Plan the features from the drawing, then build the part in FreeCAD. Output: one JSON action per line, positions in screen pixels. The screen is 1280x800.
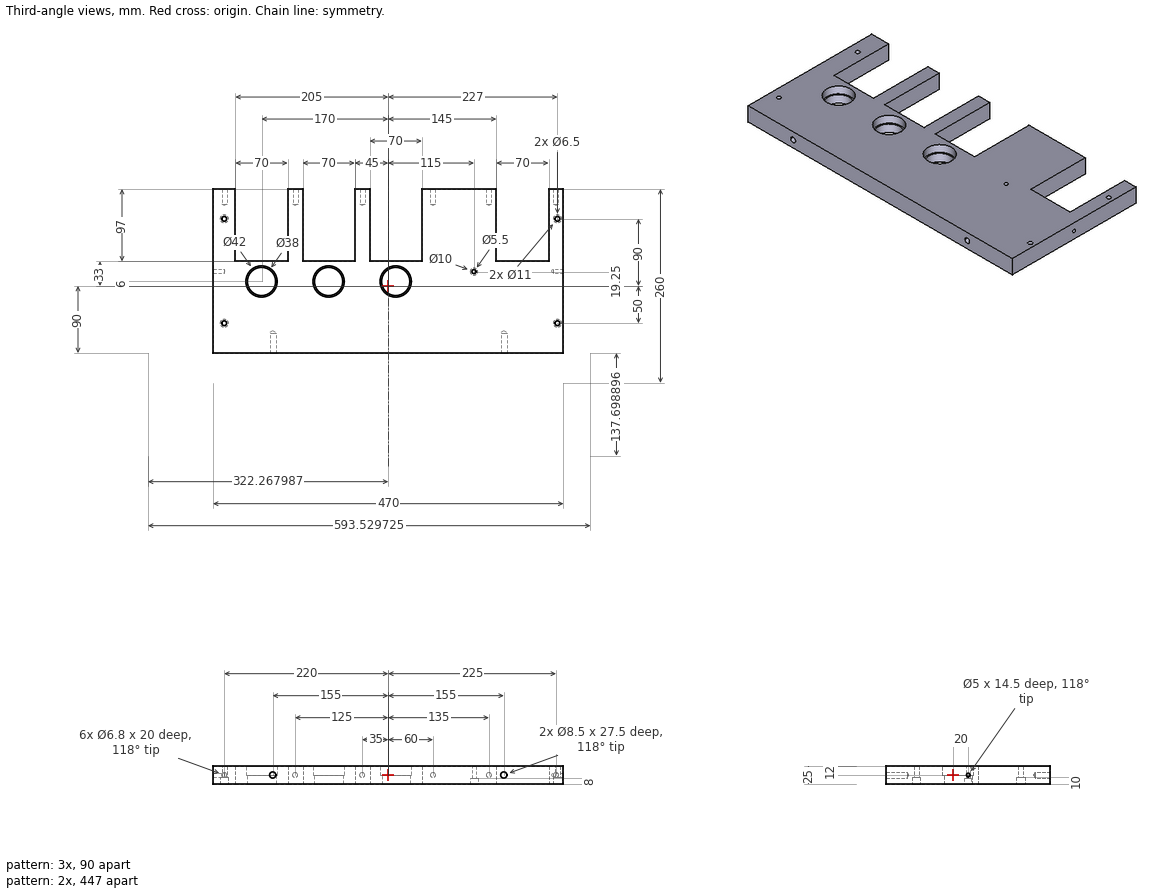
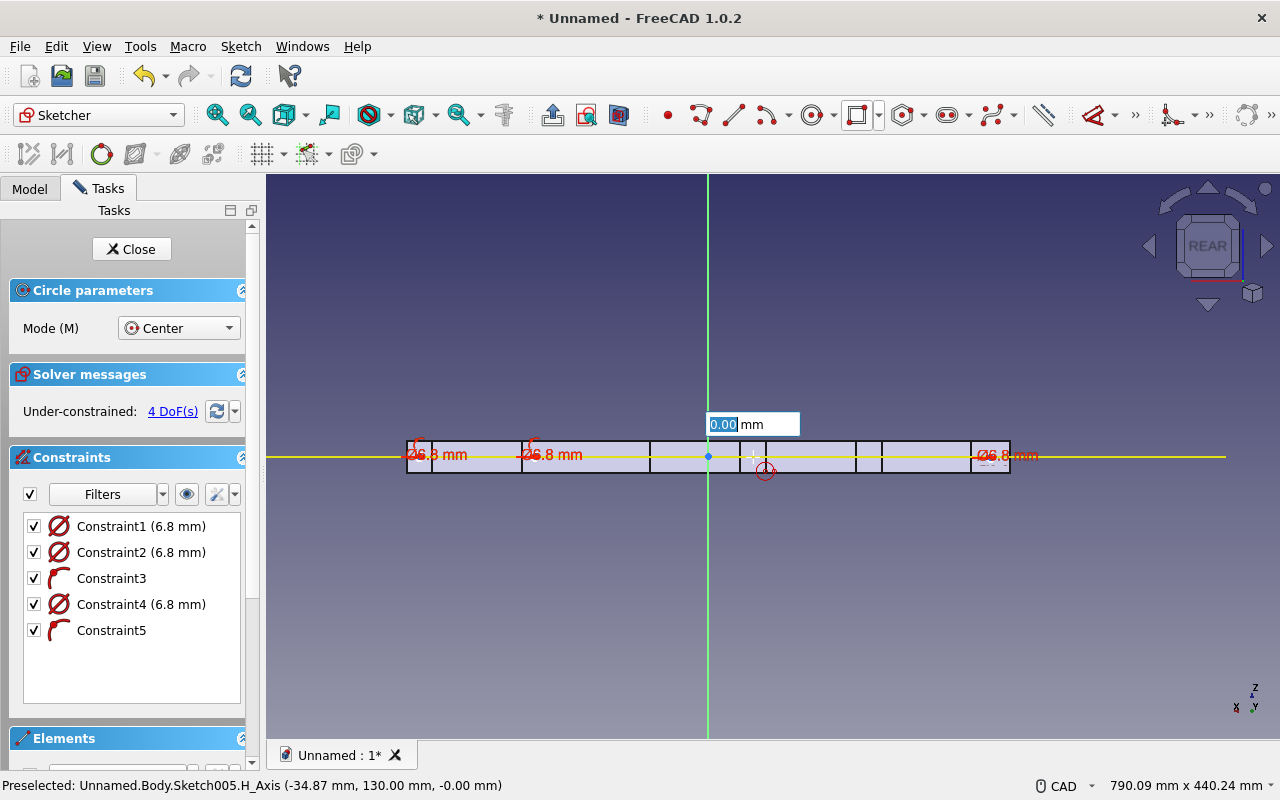
{"action": "scroll", "coordinate": [752, 461], "scroll_direction": "up", "scroll_amount": 7}
{"action": "mouse_move", "coordinate": [749, 459]}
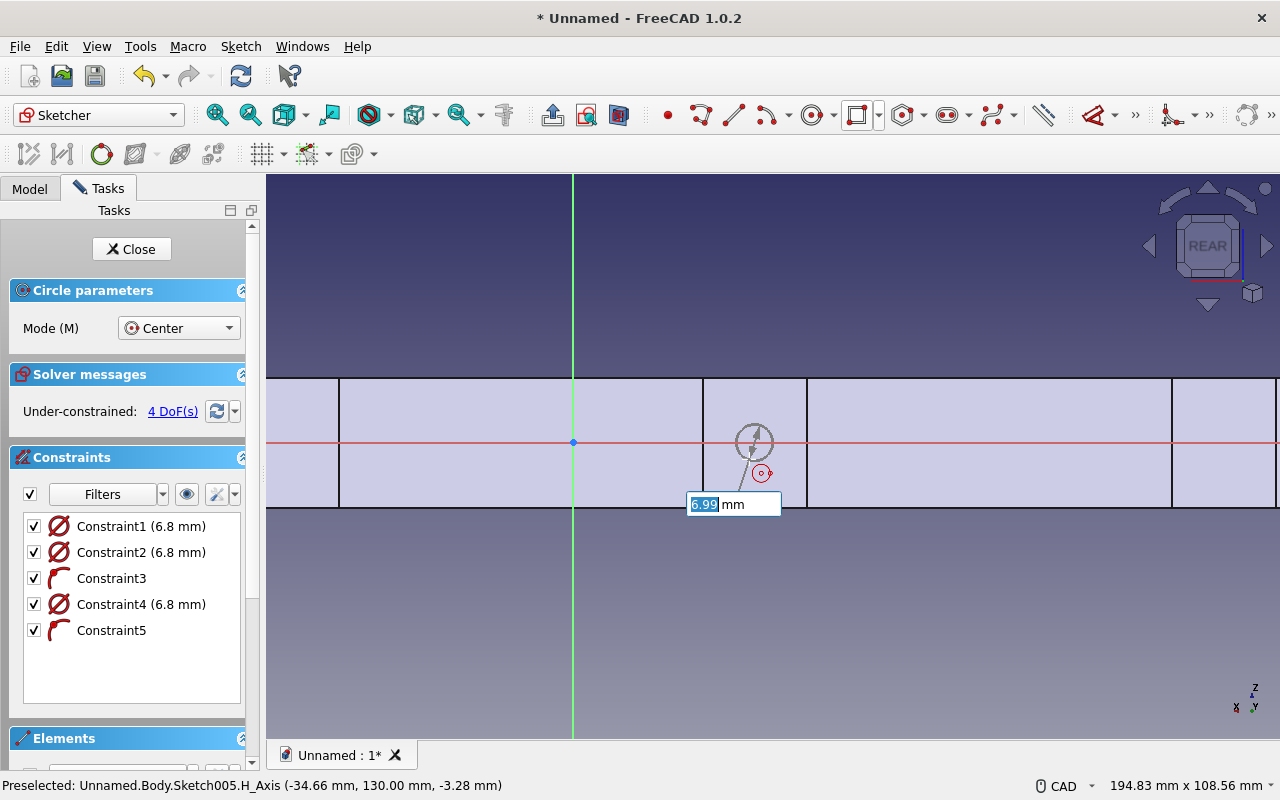
{"action": "type", "text": "6.8"}
{"action": "key", "text": "Return"}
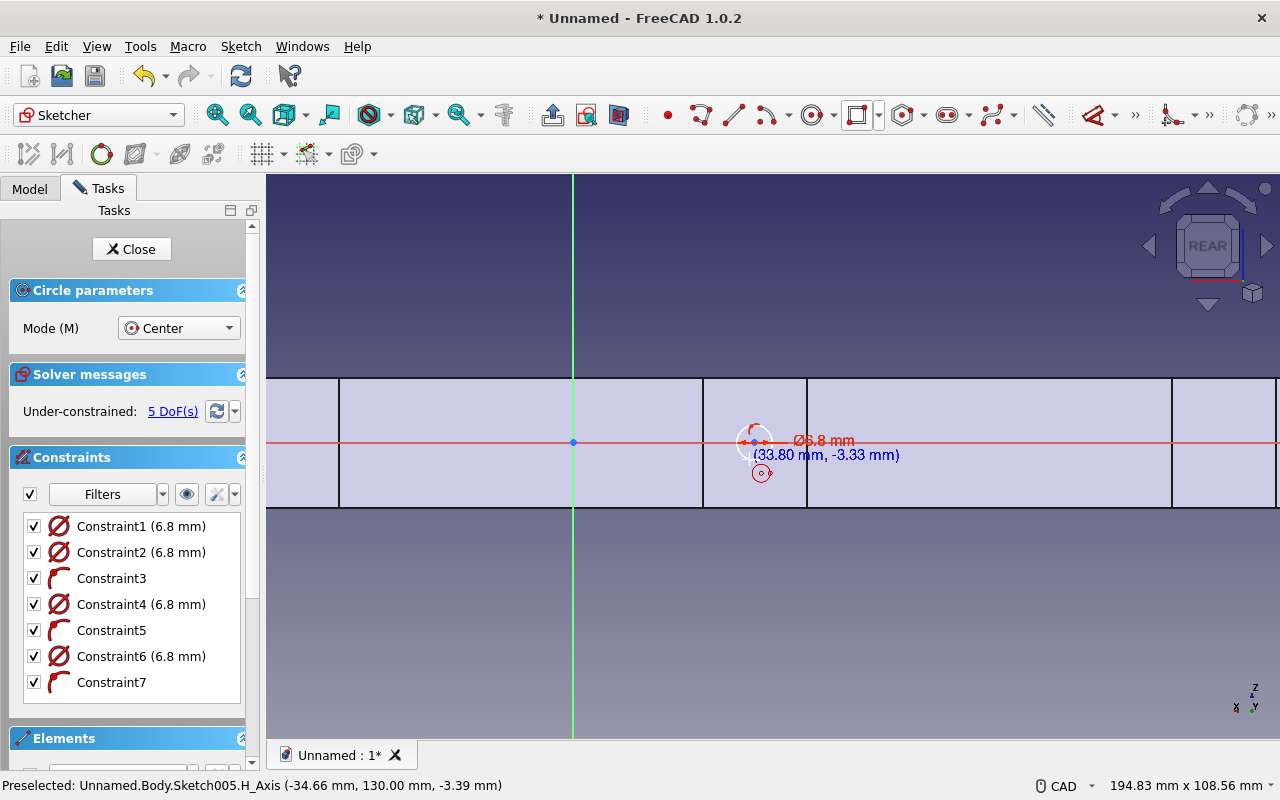
{"action": "scroll", "coordinate": [752, 461], "scroll_direction": "down", "scroll_amount": 7}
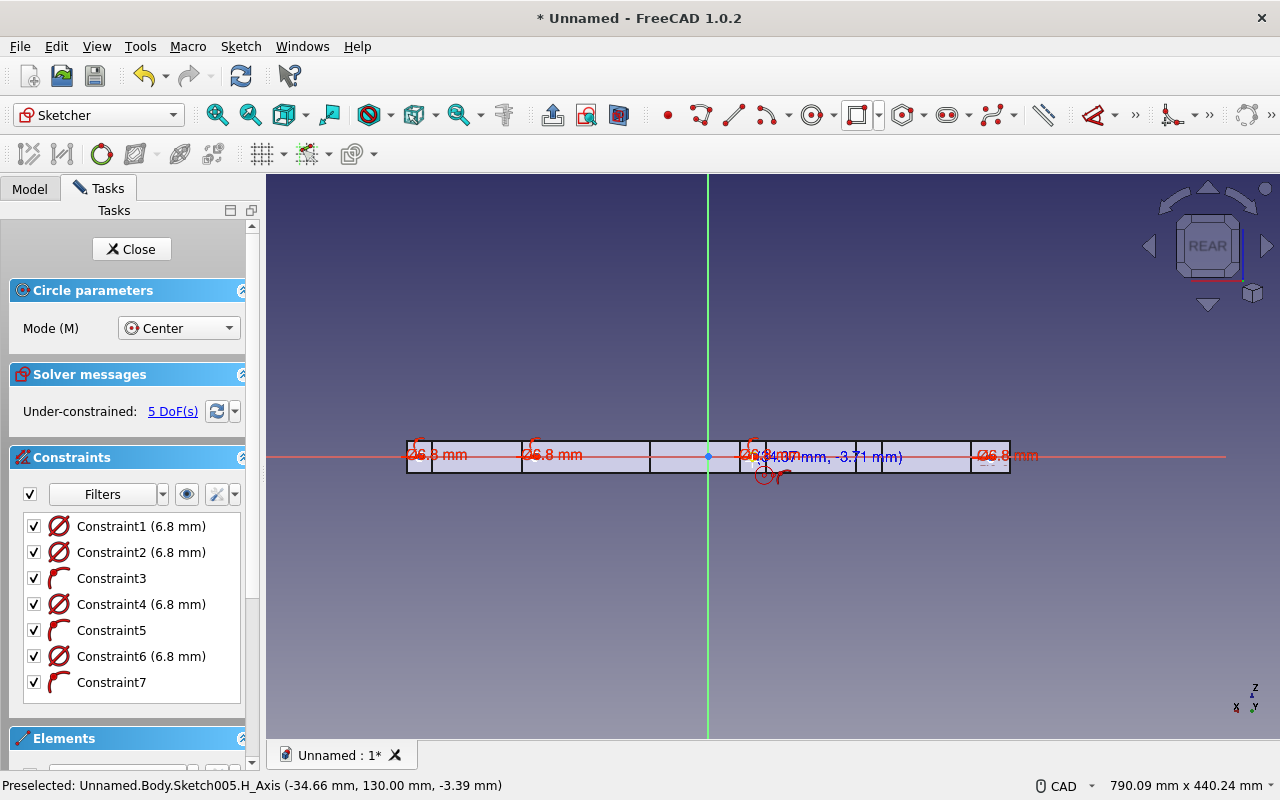
{"action": "scroll", "coordinate": [869, 457], "scroll_direction": "up", "scroll_amount": 9}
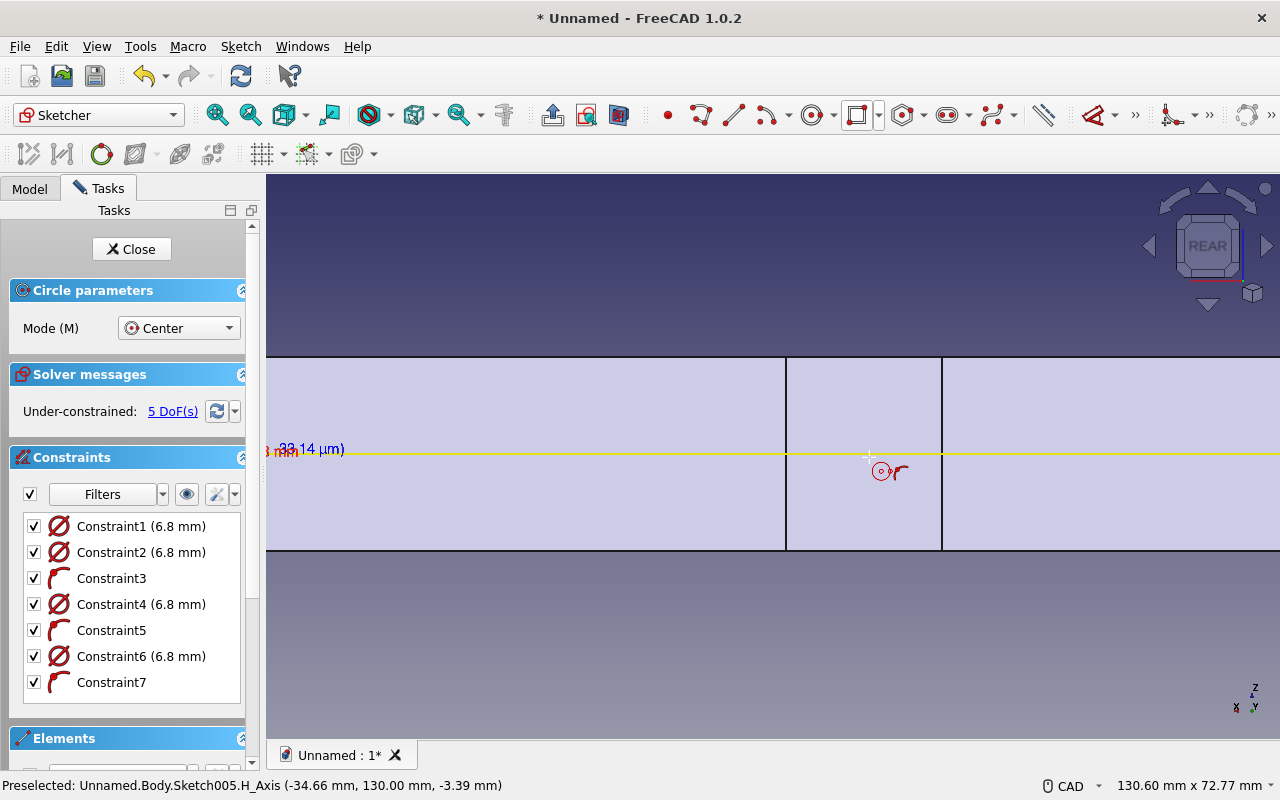
{"action": "scroll", "coordinate": [869, 457], "scroll_direction": "down", "scroll_amount": 9}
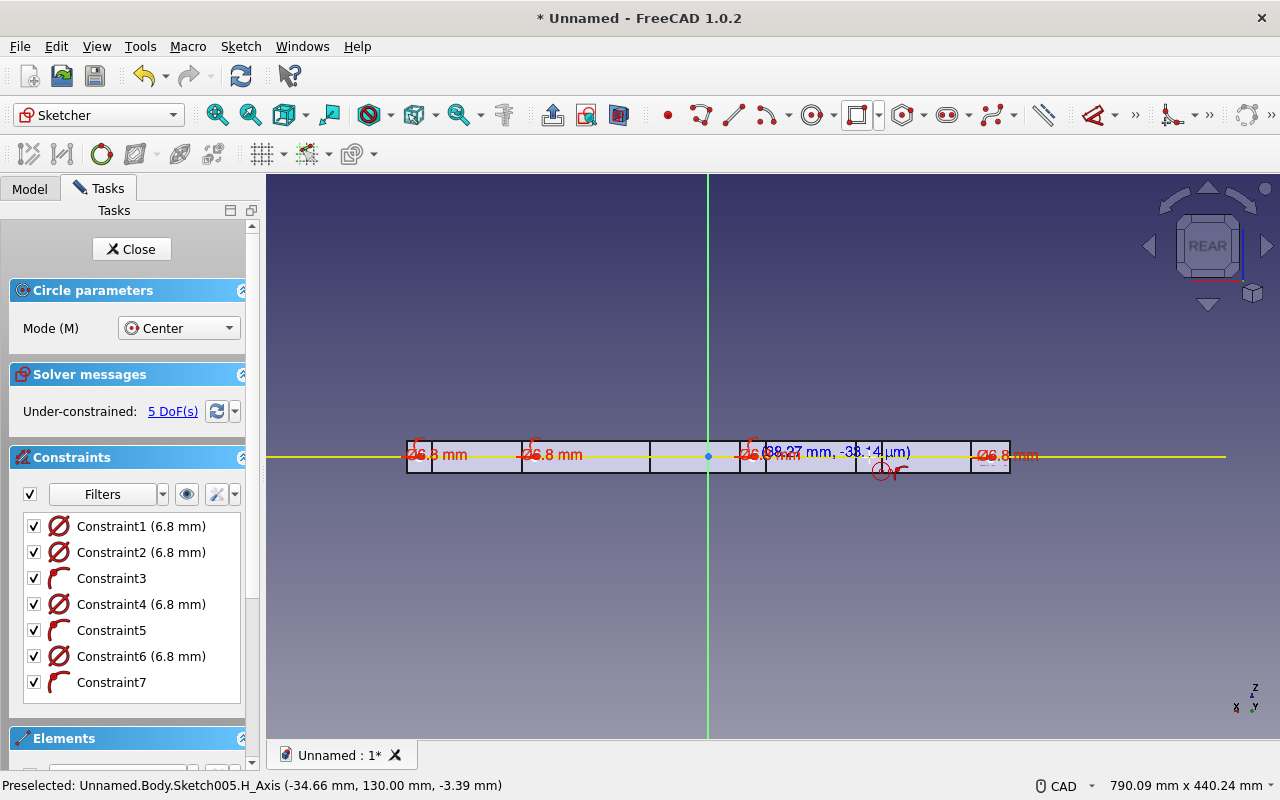
{"action": "left_click", "coordinate": [869, 457]}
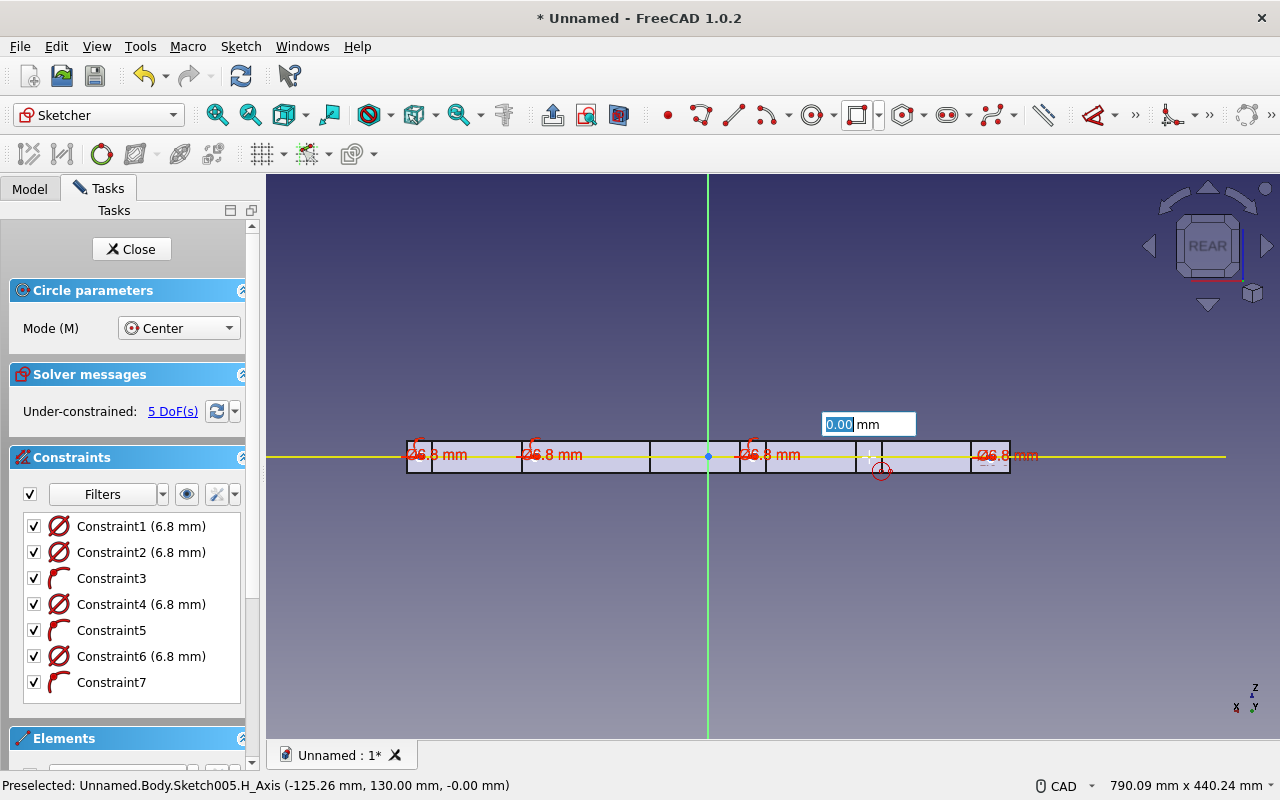
{"action": "scroll", "coordinate": [867, 461], "scroll_direction": "up", "scroll_amount": 7}
{"action": "mouse_move", "coordinate": [866, 459]}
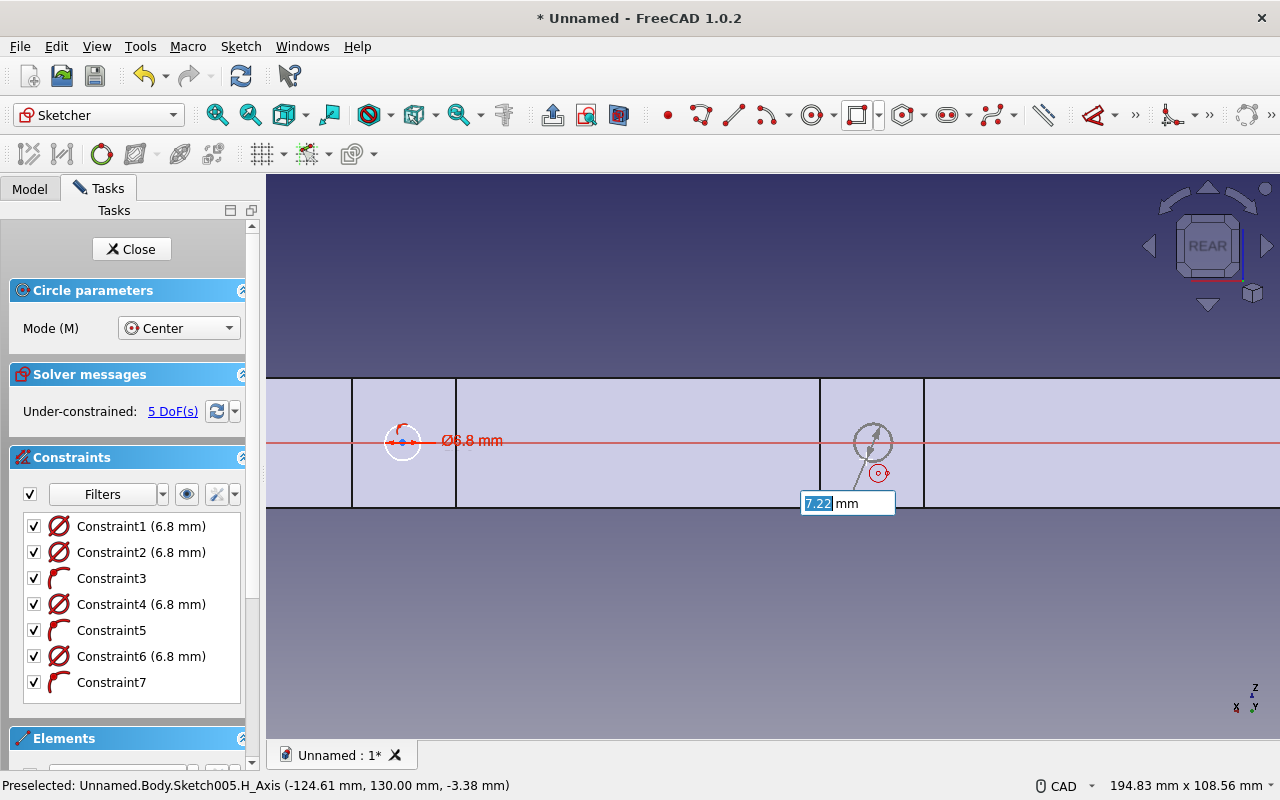
{"action": "type", "text": "6.8"}
{"action": "key", "text": "Return"}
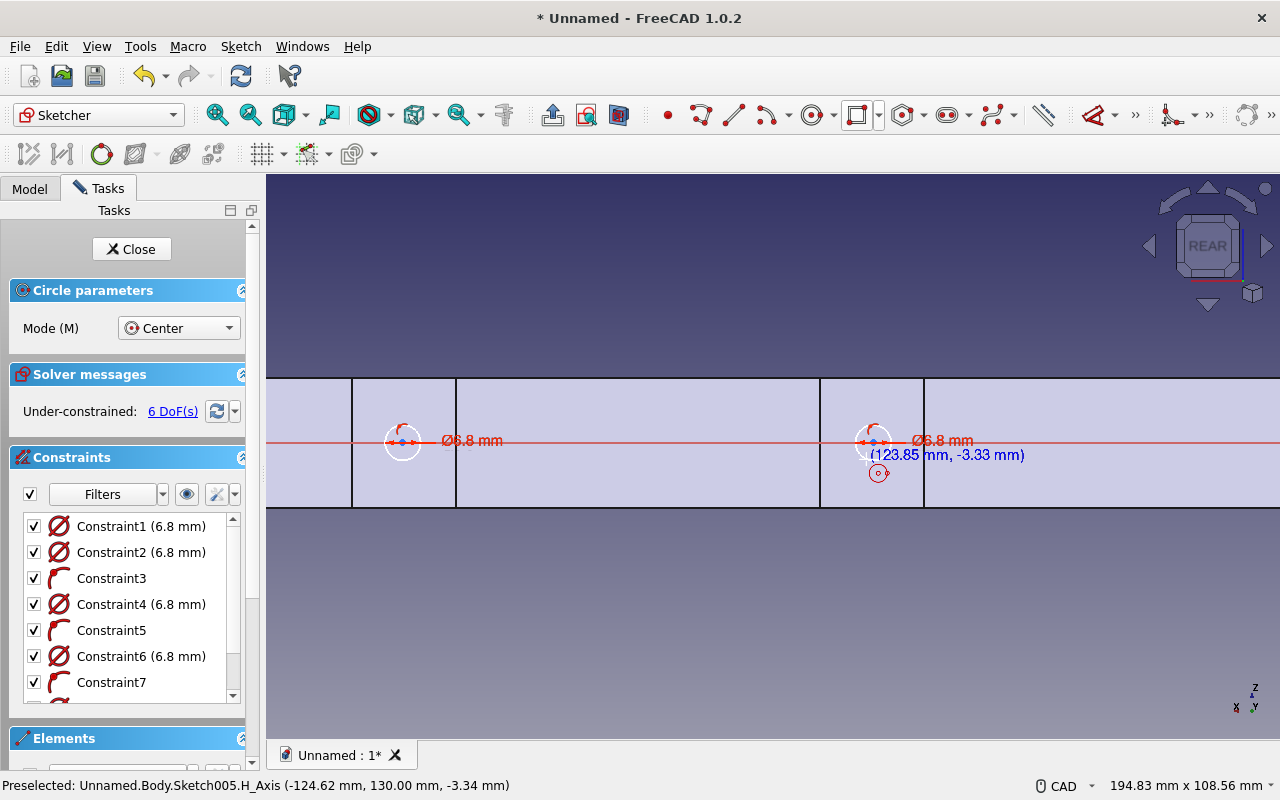
{"action": "scroll", "coordinate": [867, 461], "scroll_direction": "down", "scroll_amount": 7}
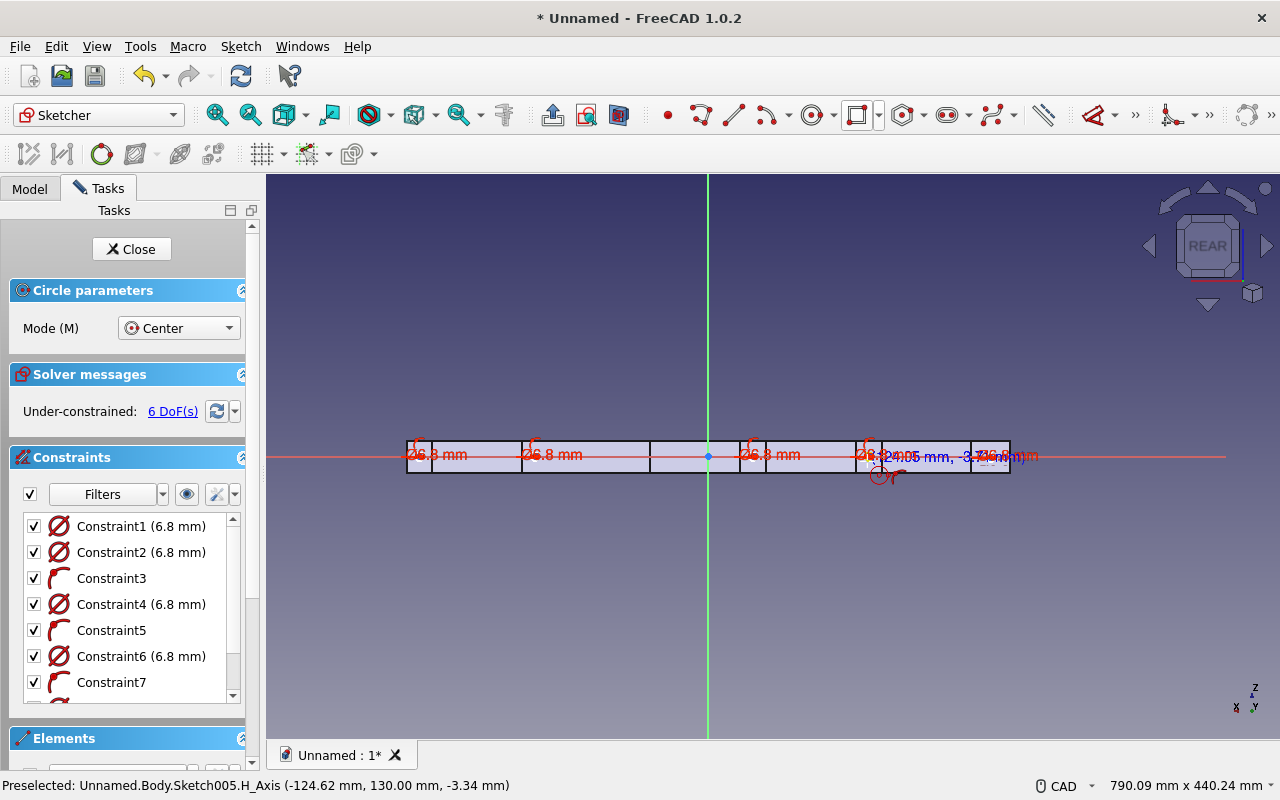
{"action": "scroll", "coordinate": [631, 457], "scroll_direction": "up", "scroll_amount": 9}